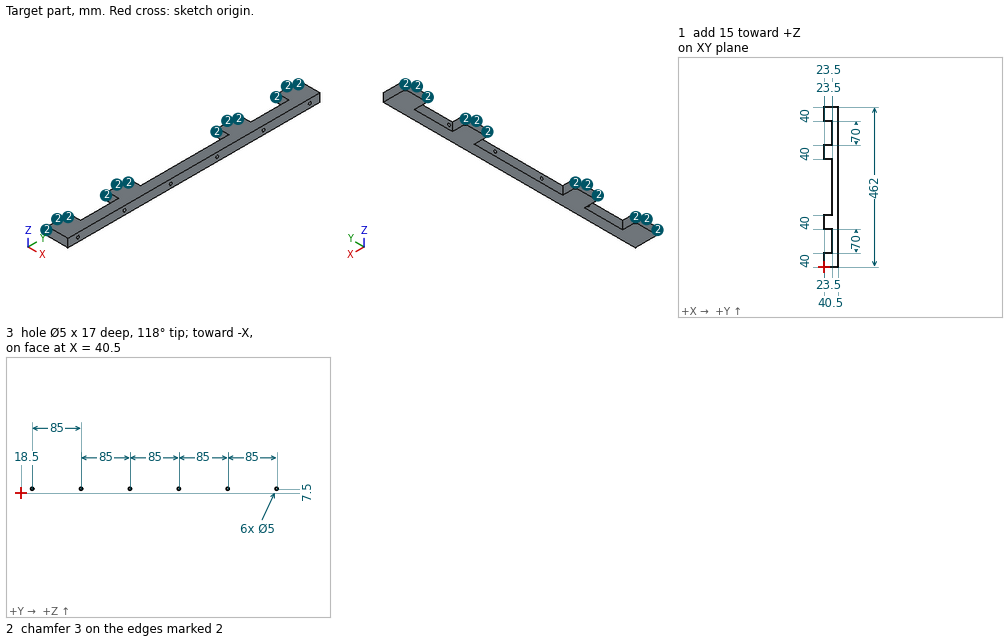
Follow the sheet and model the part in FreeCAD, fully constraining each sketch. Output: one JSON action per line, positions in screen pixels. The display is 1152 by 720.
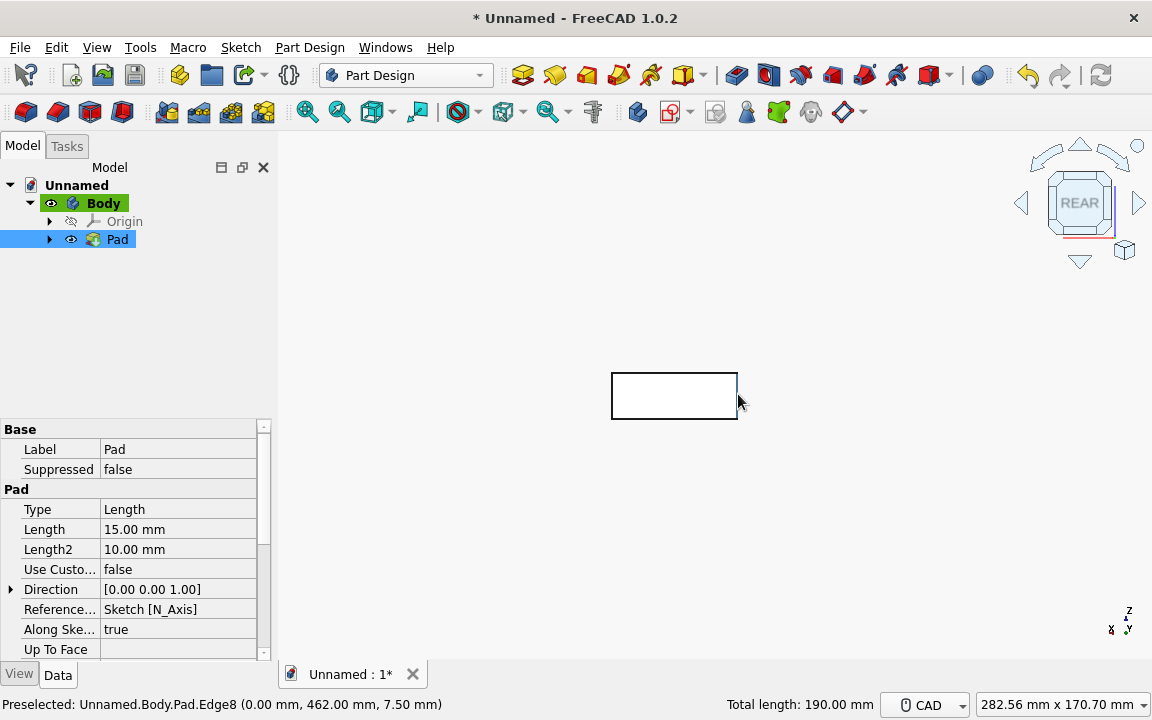
{"action": "left_click", "coordinate": [308, 112]}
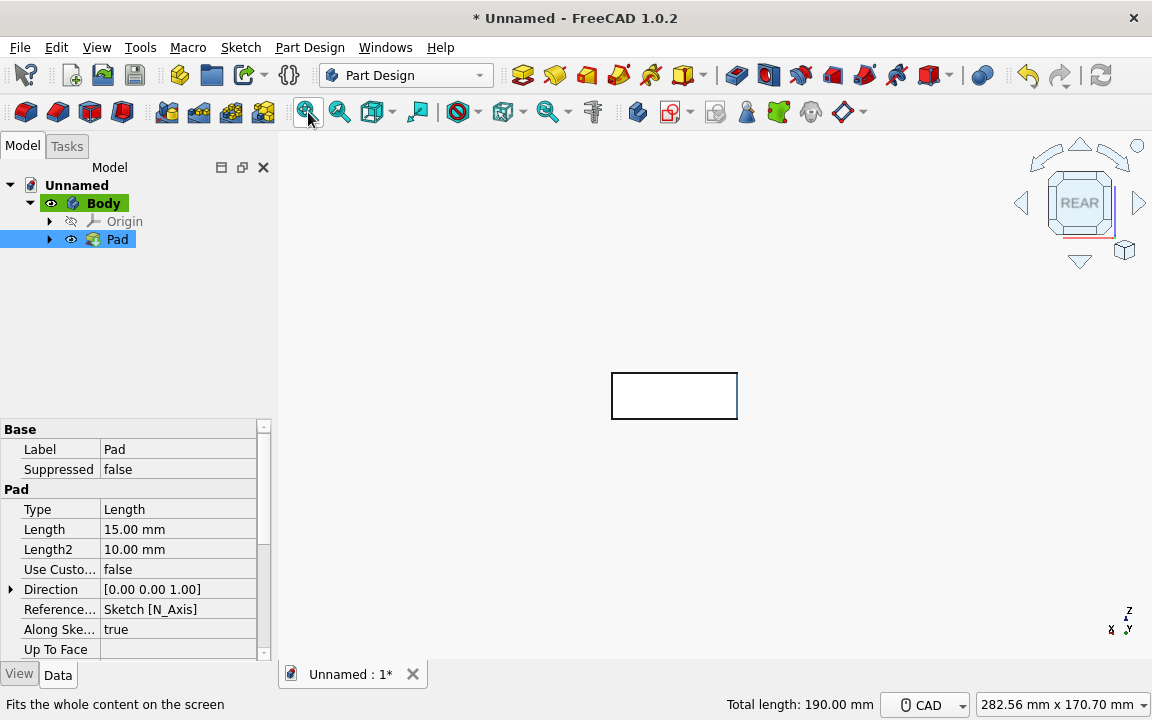
{"action": "key", "text": "6"}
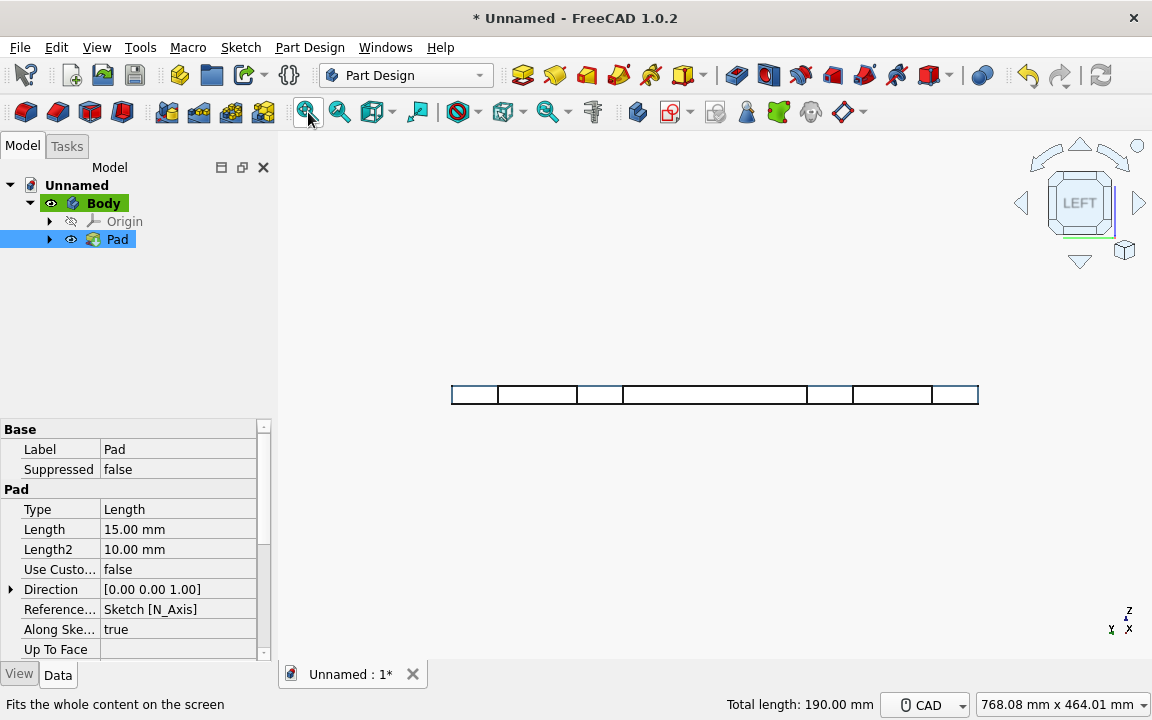
{"action": "left_click", "coordinate": [853, 394], "text": "ctrl"}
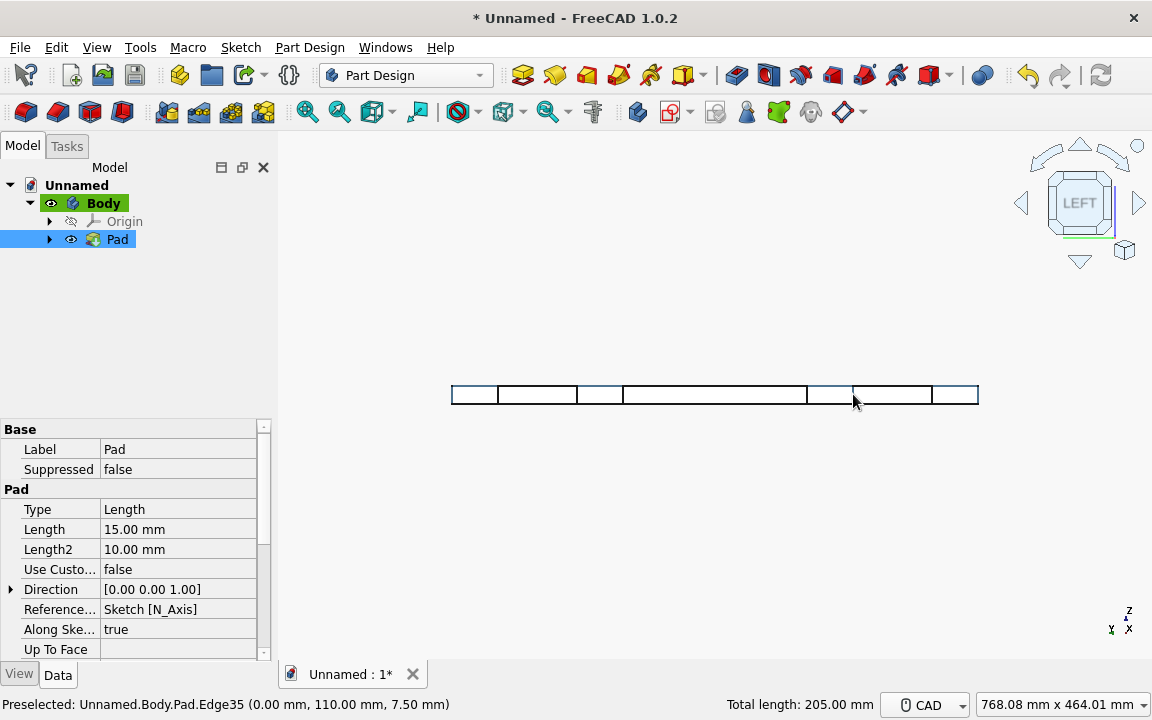
{"action": "left_click", "coordinate": [807, 394], "text": "ctrl"}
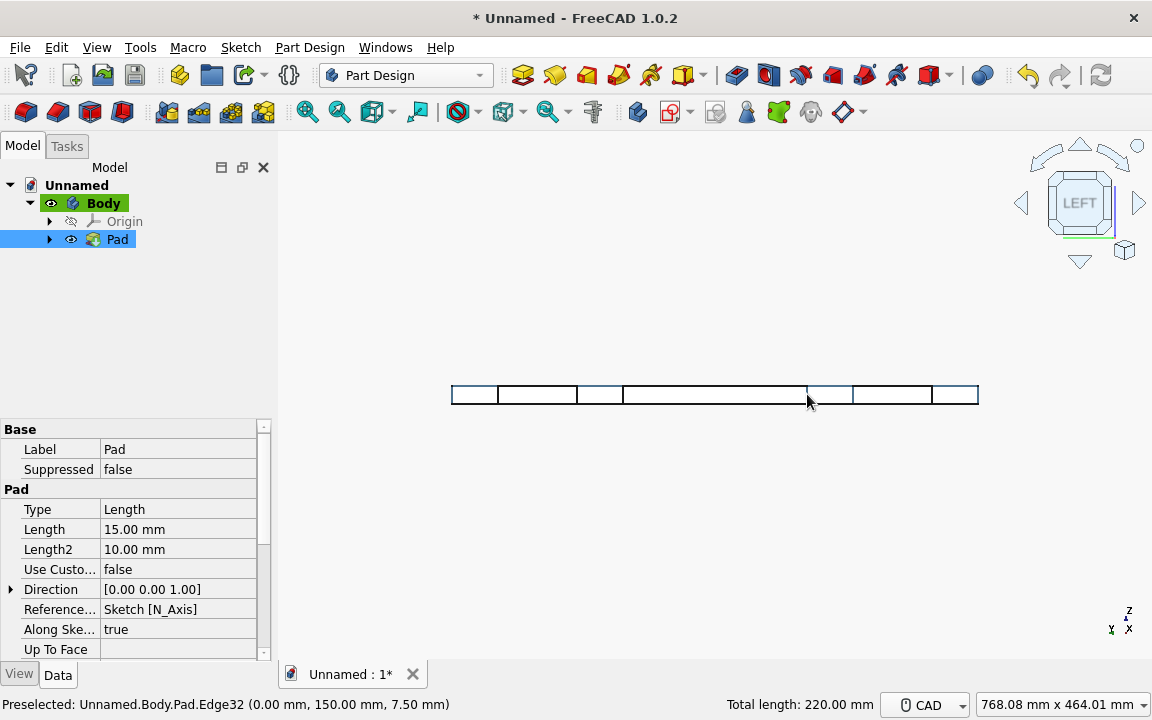
{"action": "left_click", "coordinate": [623, 394], "text": "ctrl"}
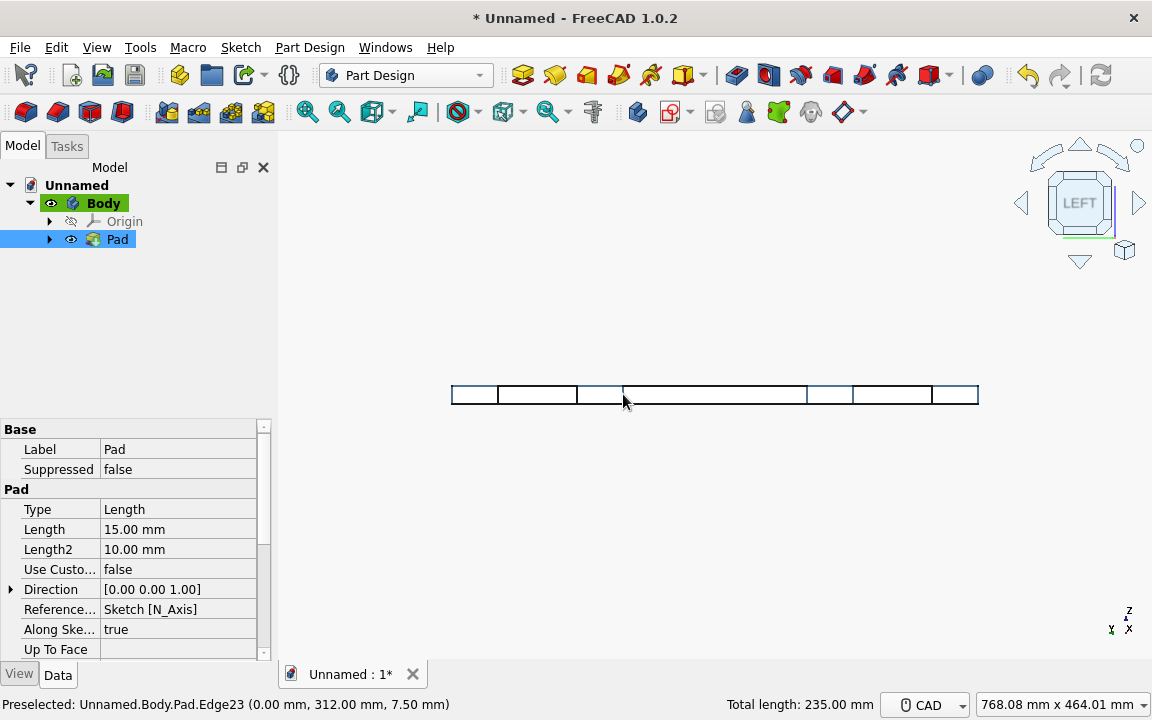
{"action": "left_click", "coordinate": [577, 394], "text": "ctrl"}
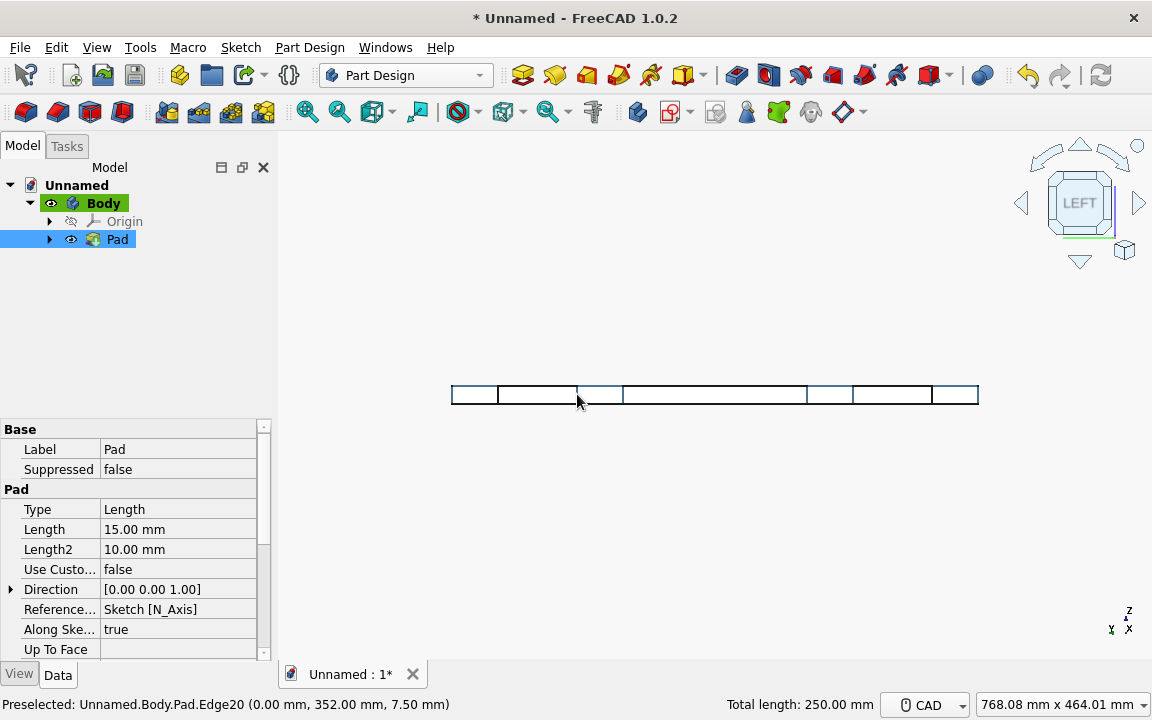
{"action": "left_click", "coordinate": [498, 394], "text": "ctrl"}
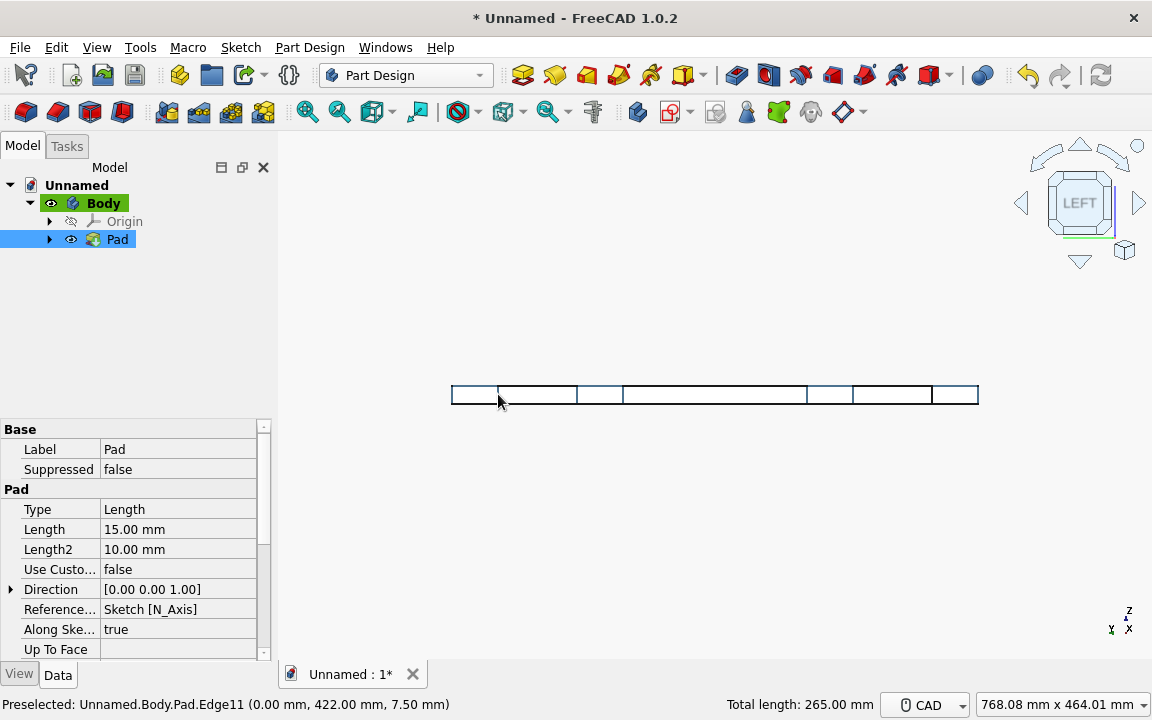
{"action": "left_click", "coordinate": [932, 394], "text": "ctrl"}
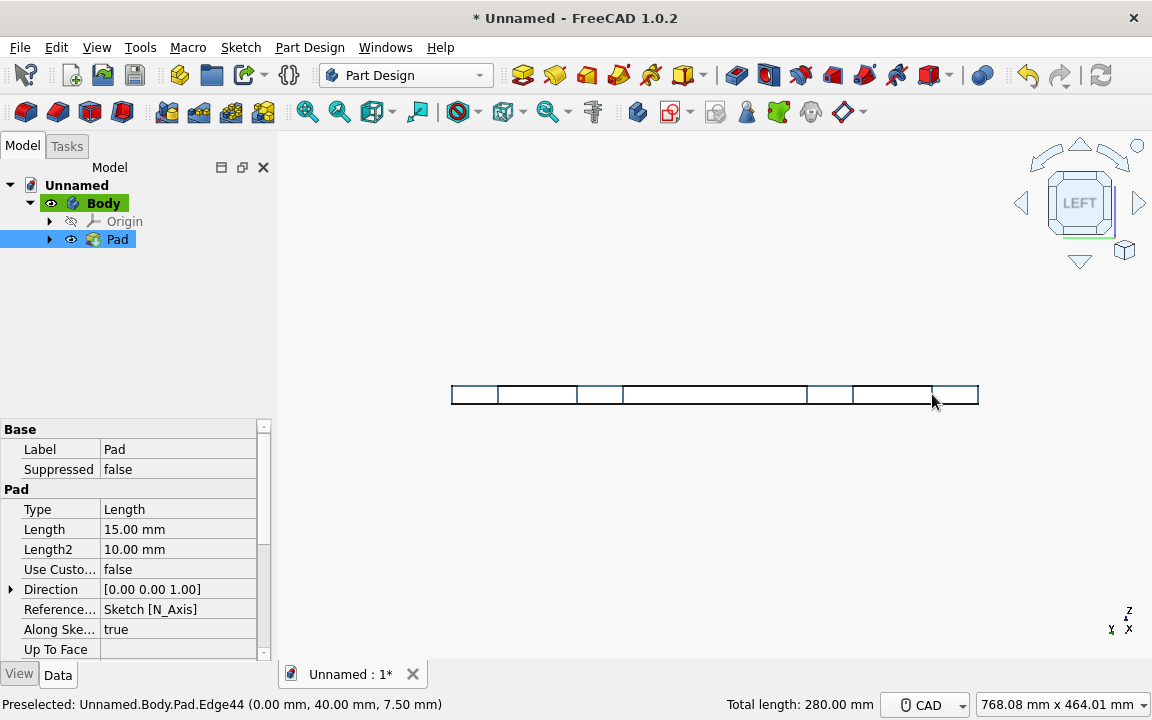
{"action": "left_click", "coordinate": [58, 112]}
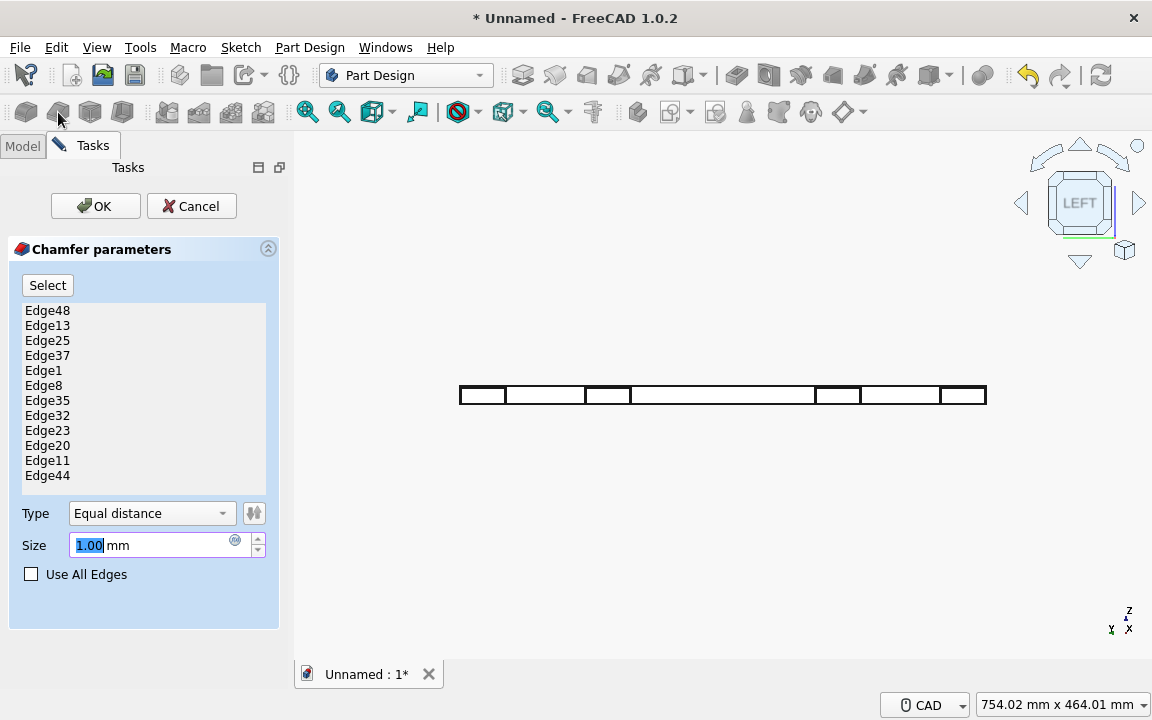
{"action": "type", "text": "3"}
{"action": "key", "text": "Tab"}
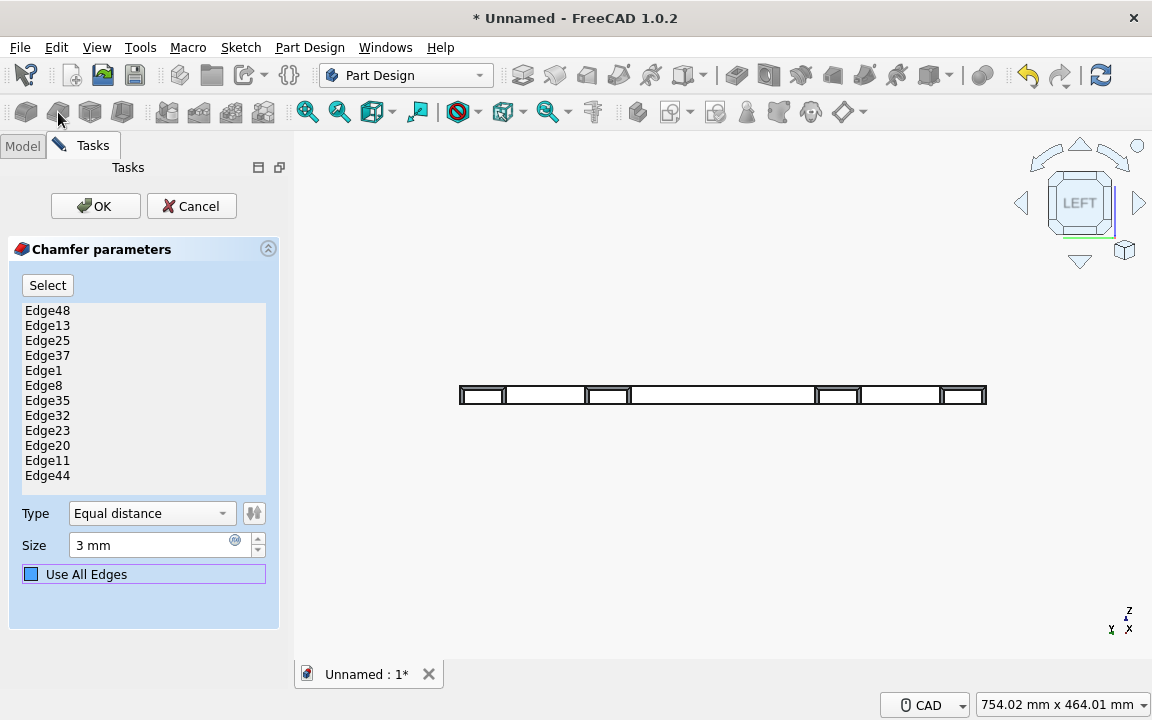
{"action": "left_click", "coordinate": [96, 206]}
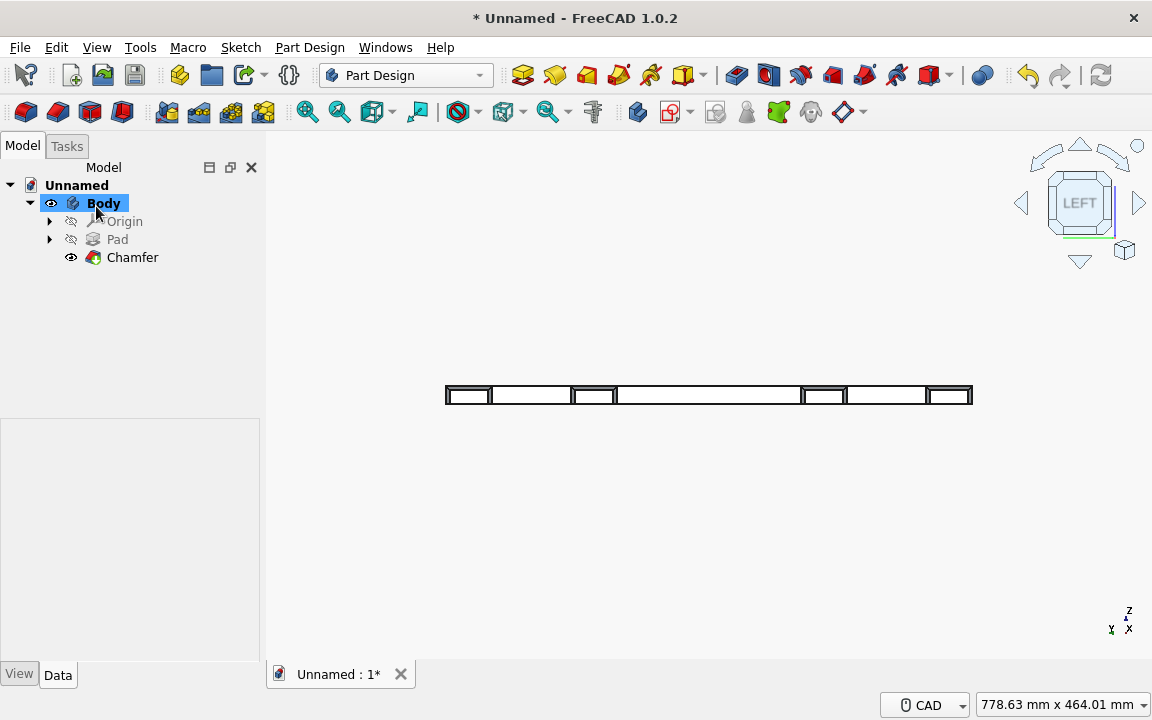
{"action": "key", "text": "0"}